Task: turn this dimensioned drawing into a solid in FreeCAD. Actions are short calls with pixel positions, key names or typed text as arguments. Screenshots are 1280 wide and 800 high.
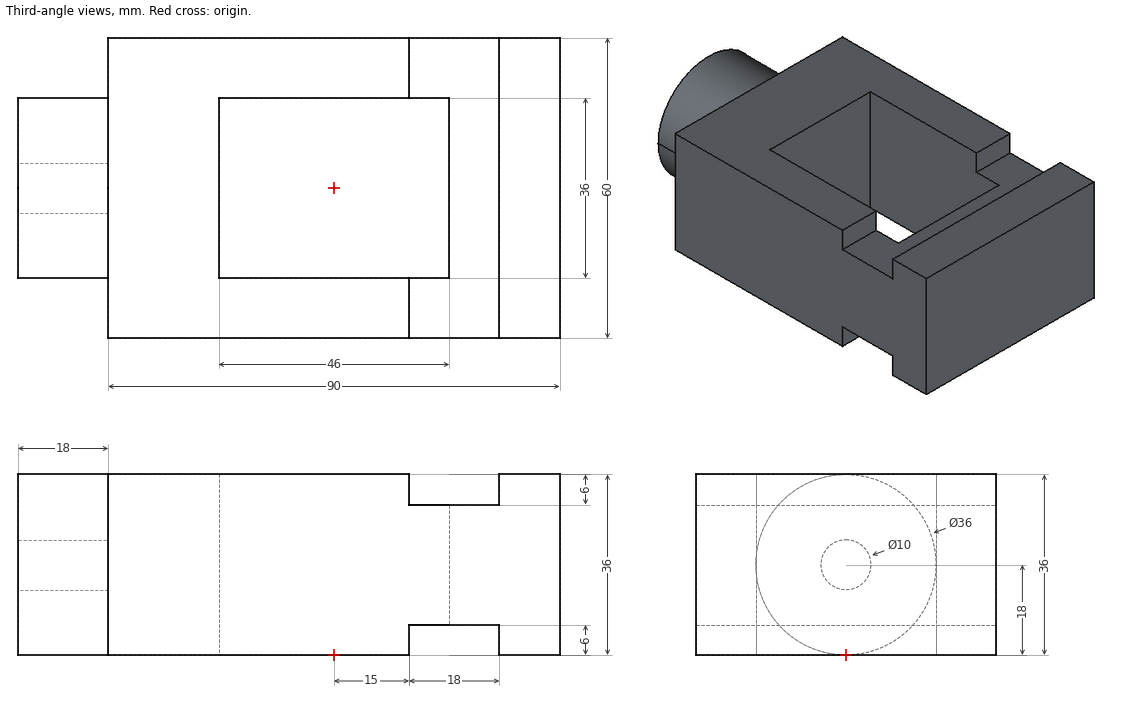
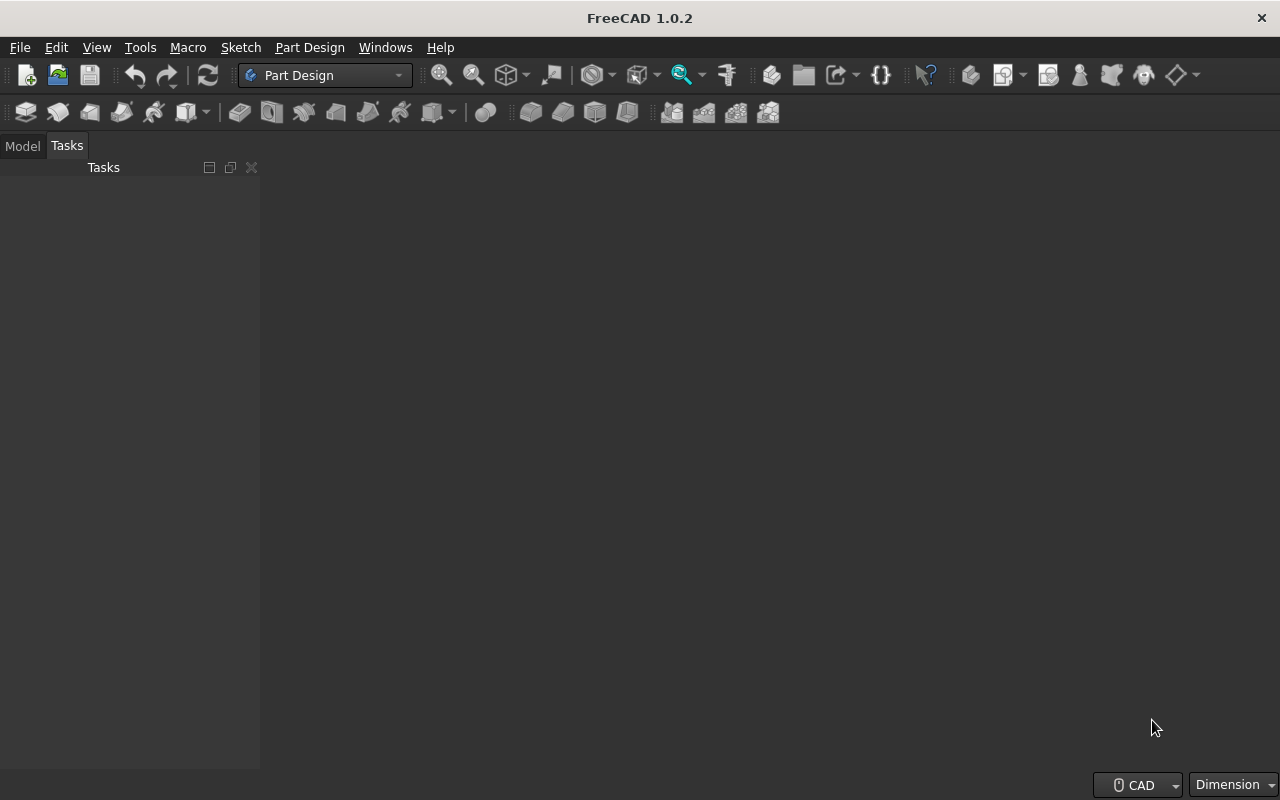
click(26, 76)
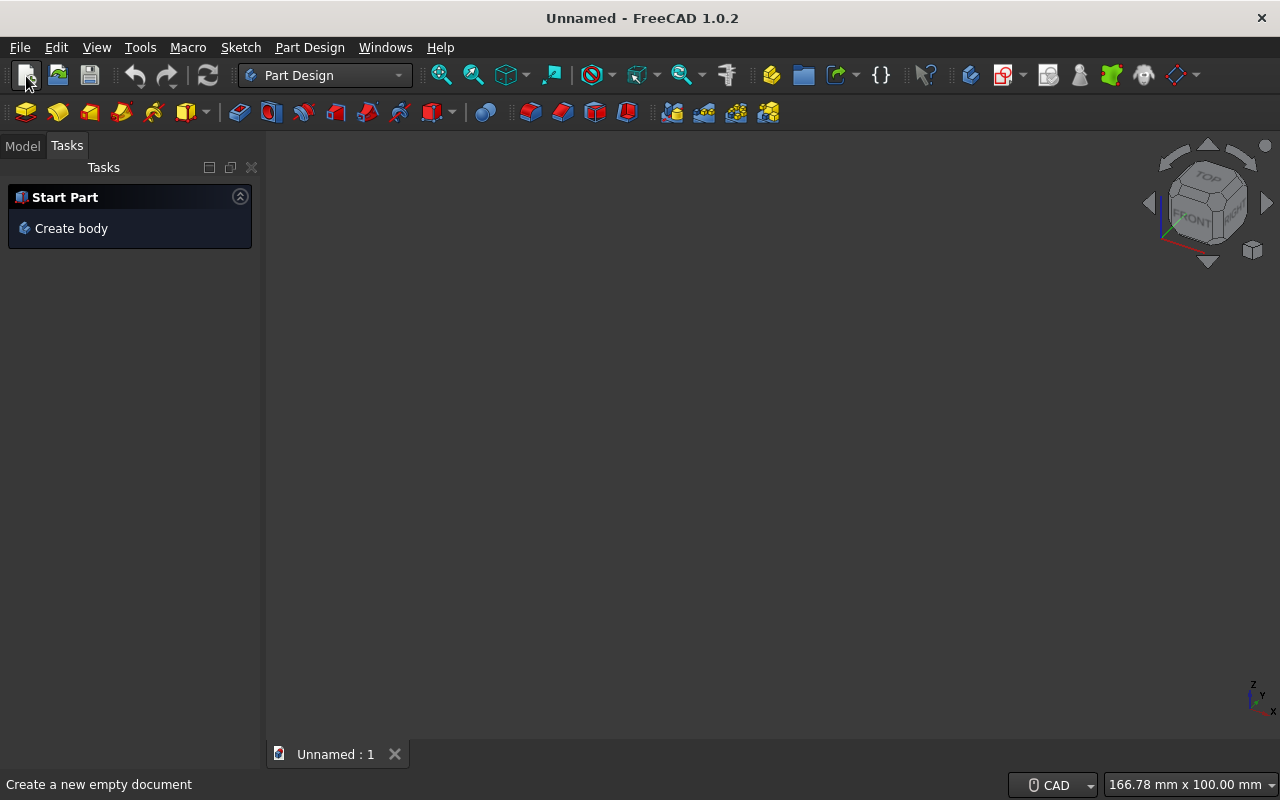
click(1004, 76)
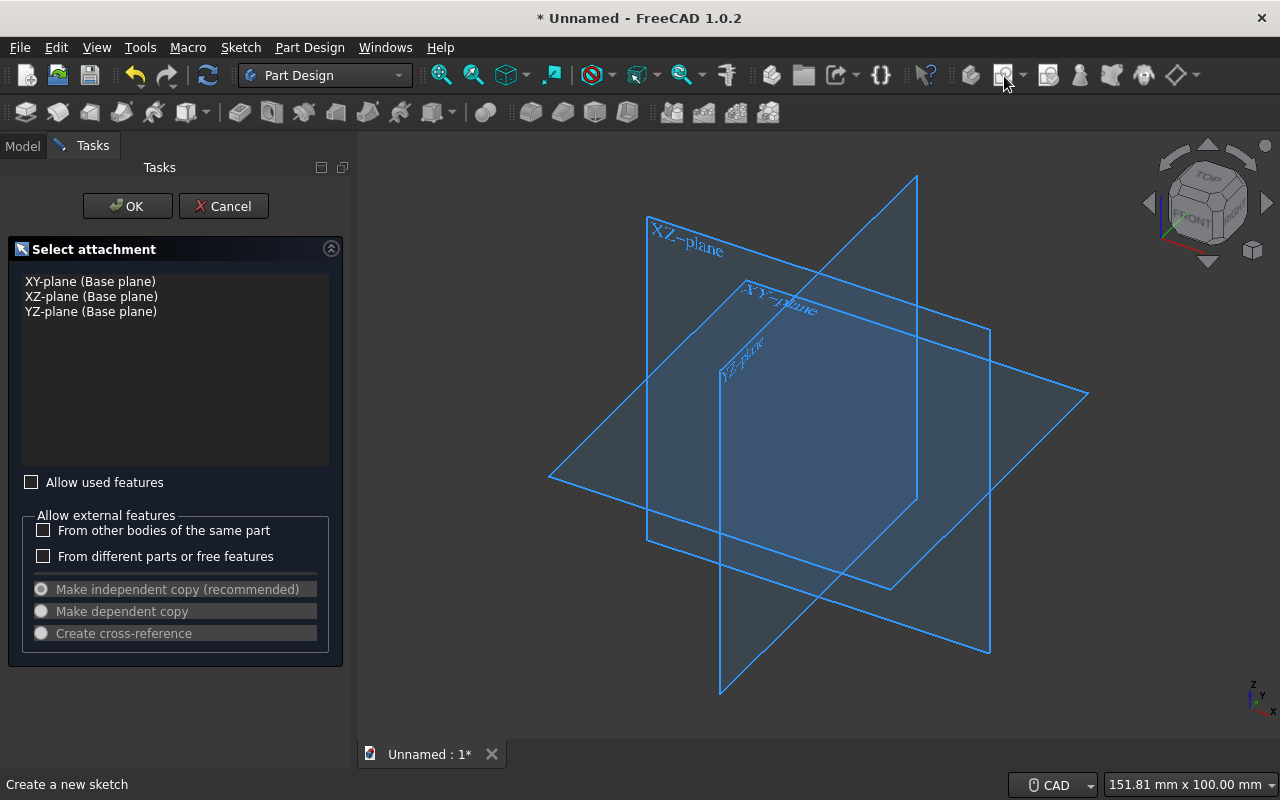
click(82, 282)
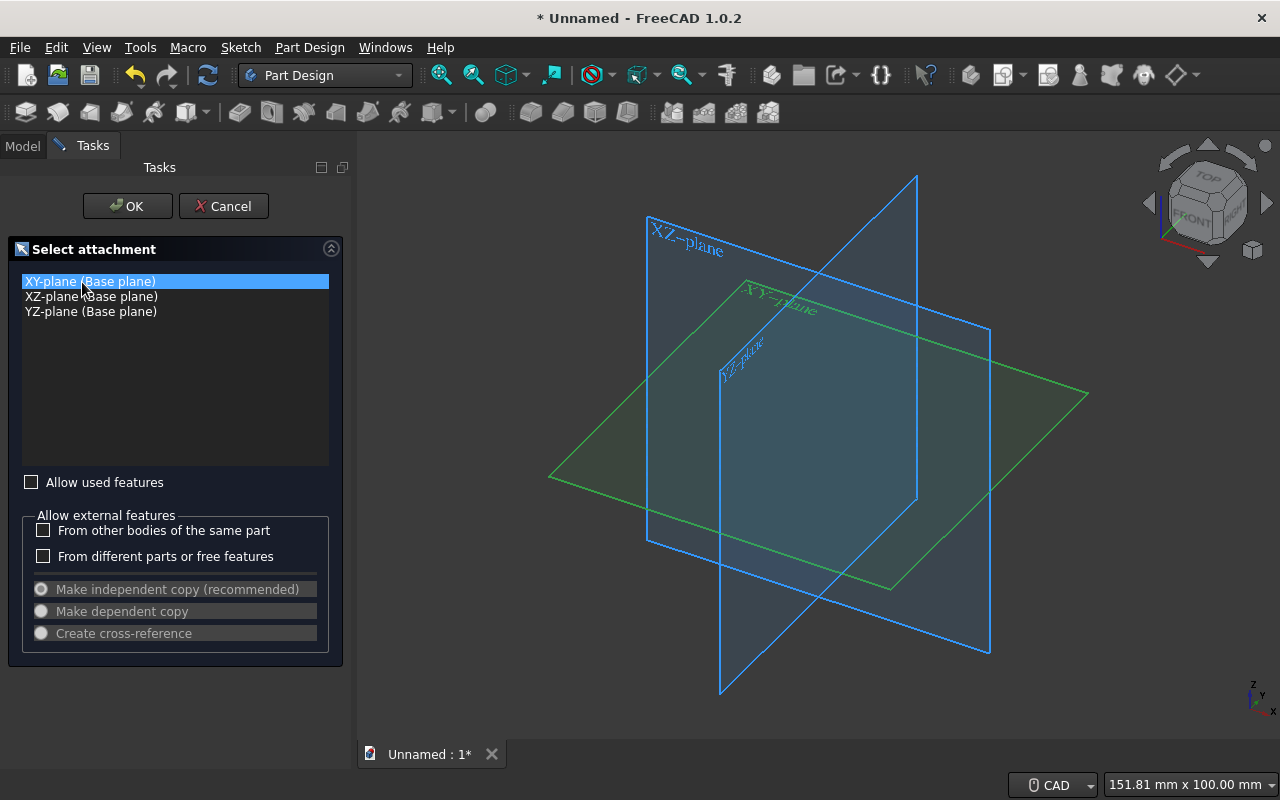
click(128, 206)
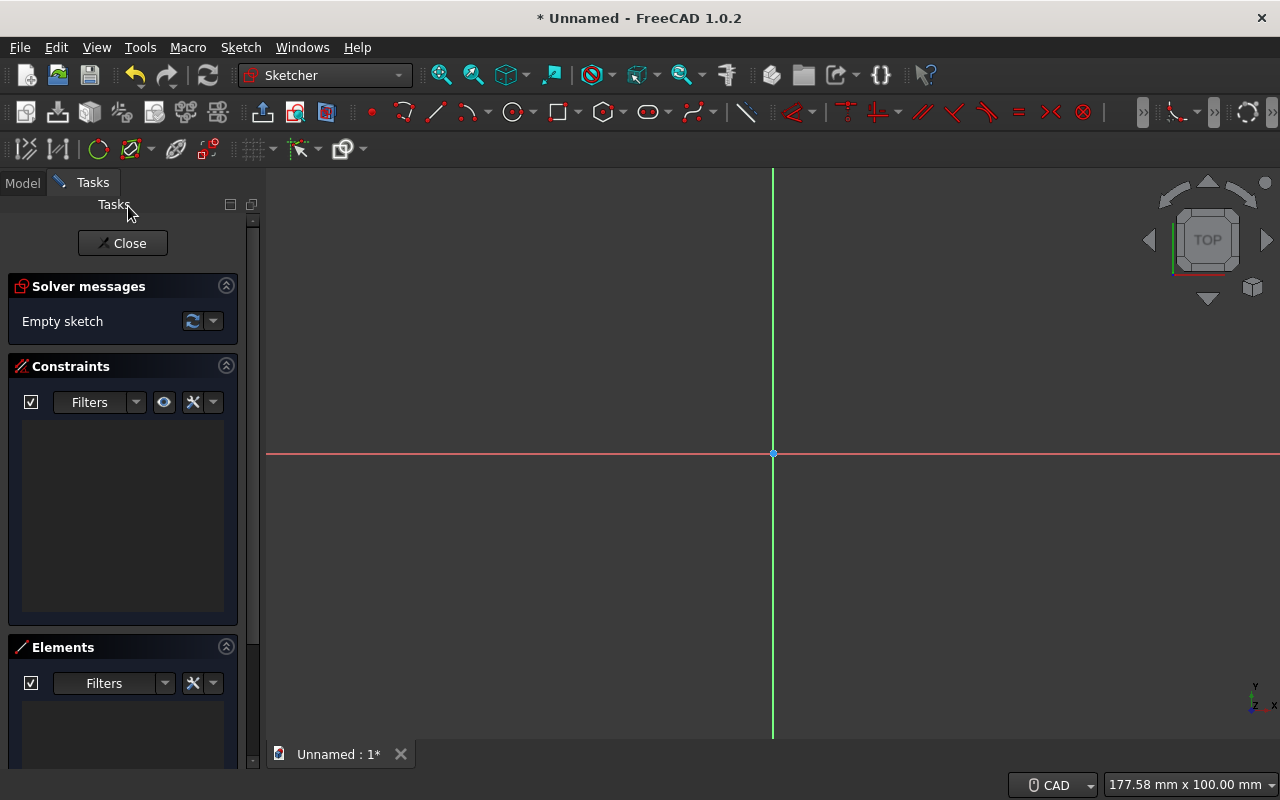
click(580, 112)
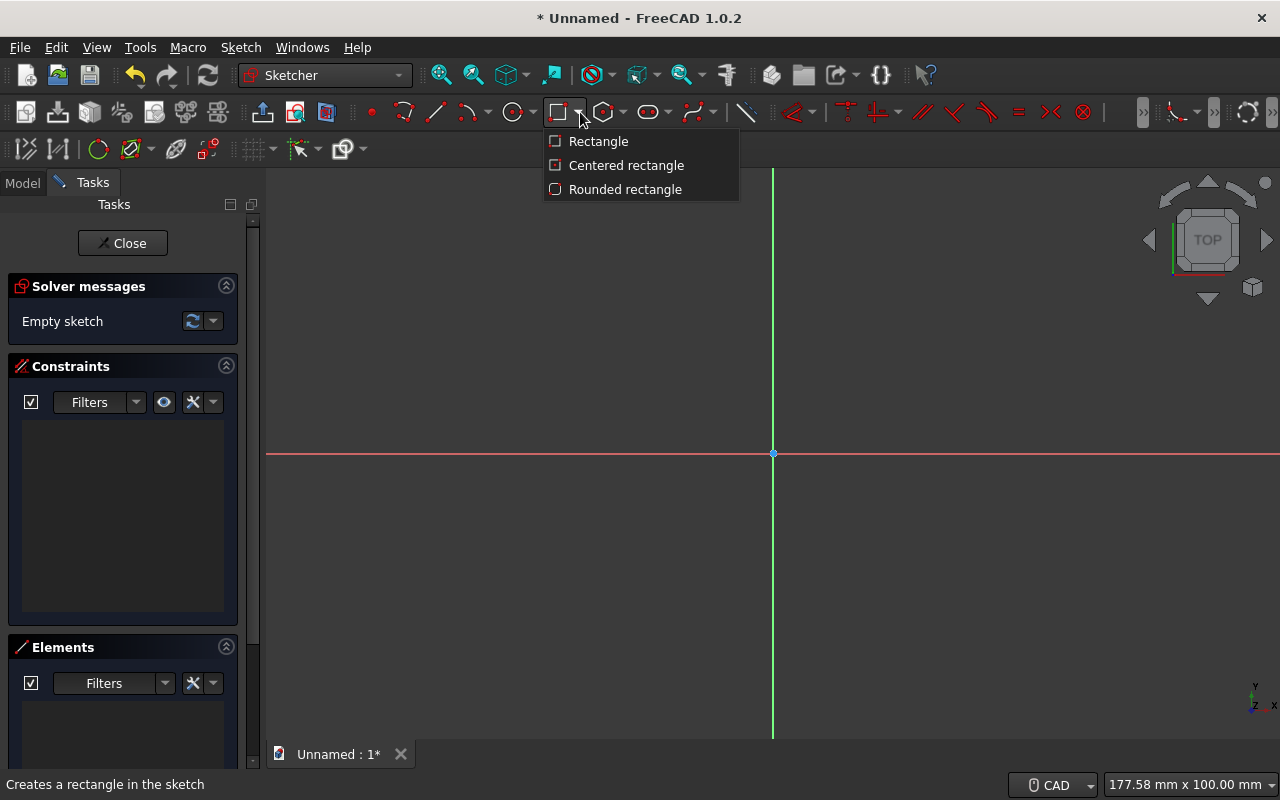
click(642, 165)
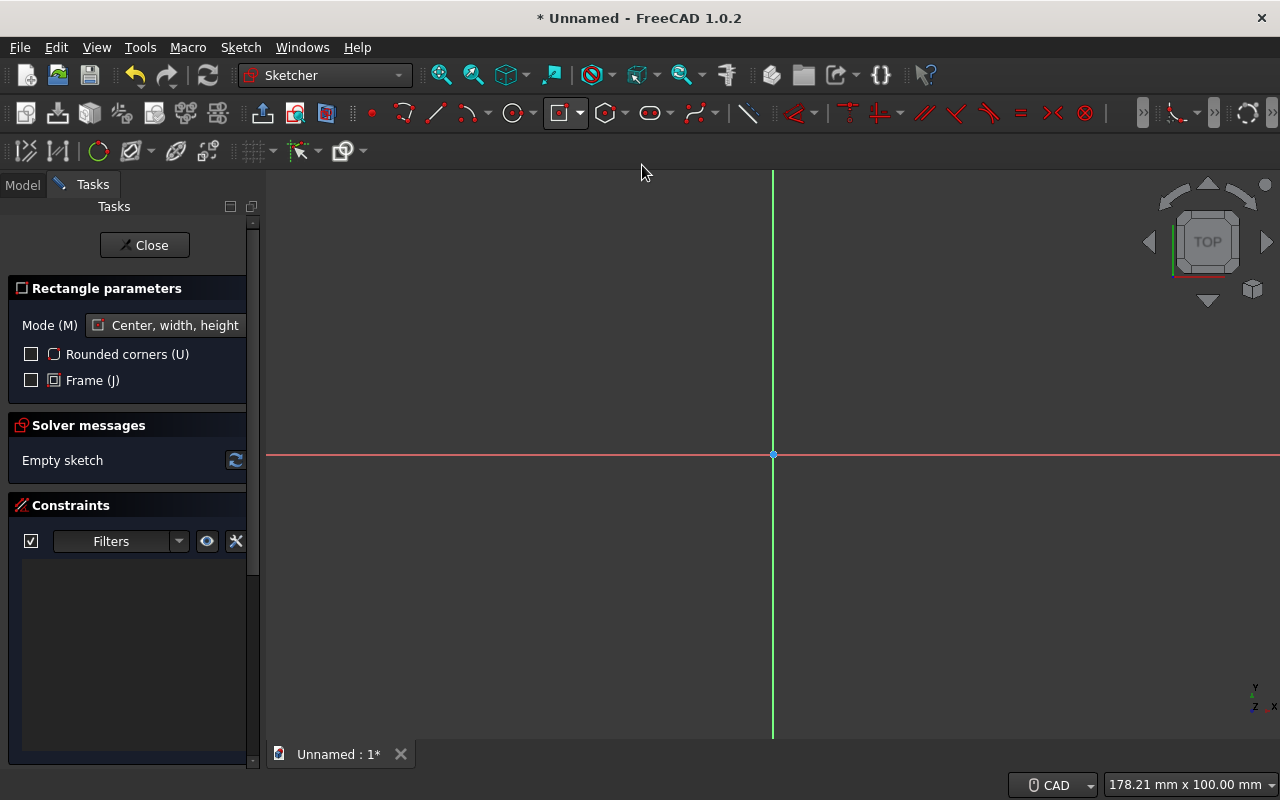
click(773, 454)
click(1029, 284)
key(Escape)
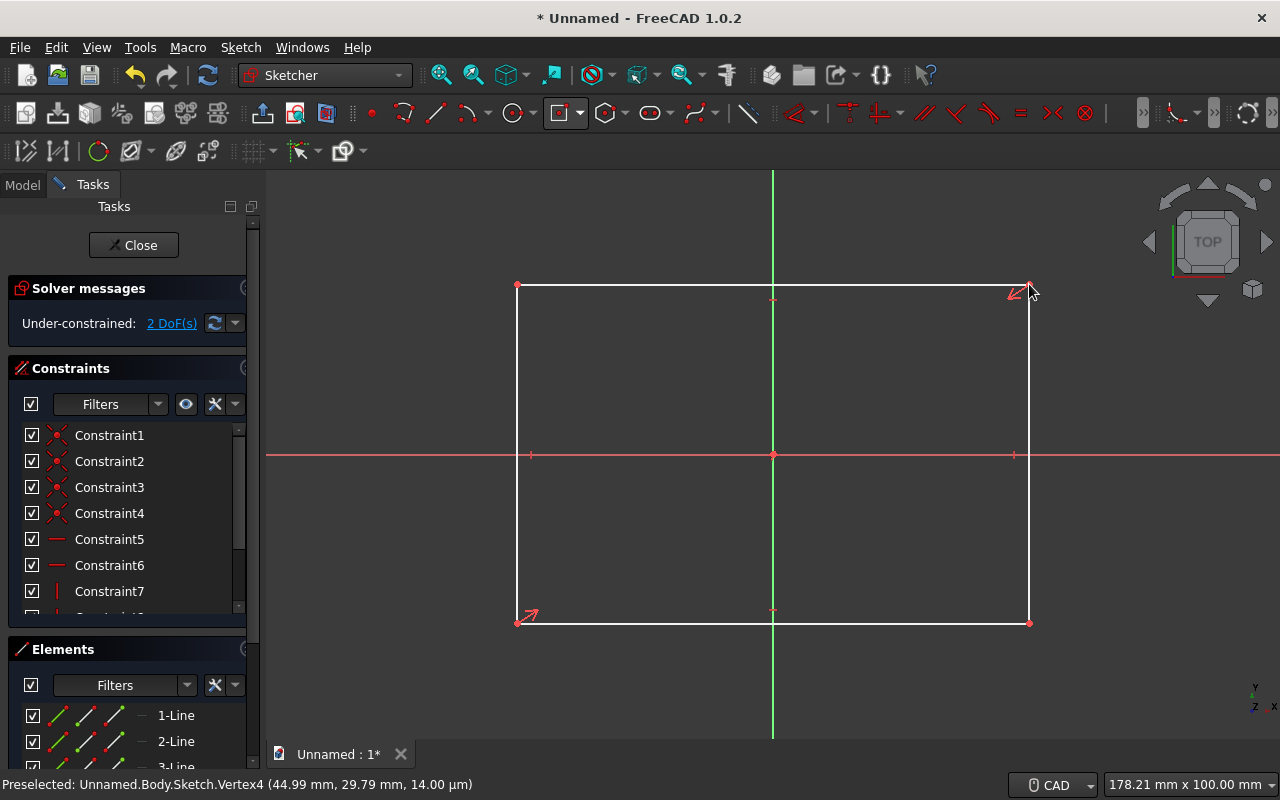
click(671, 624)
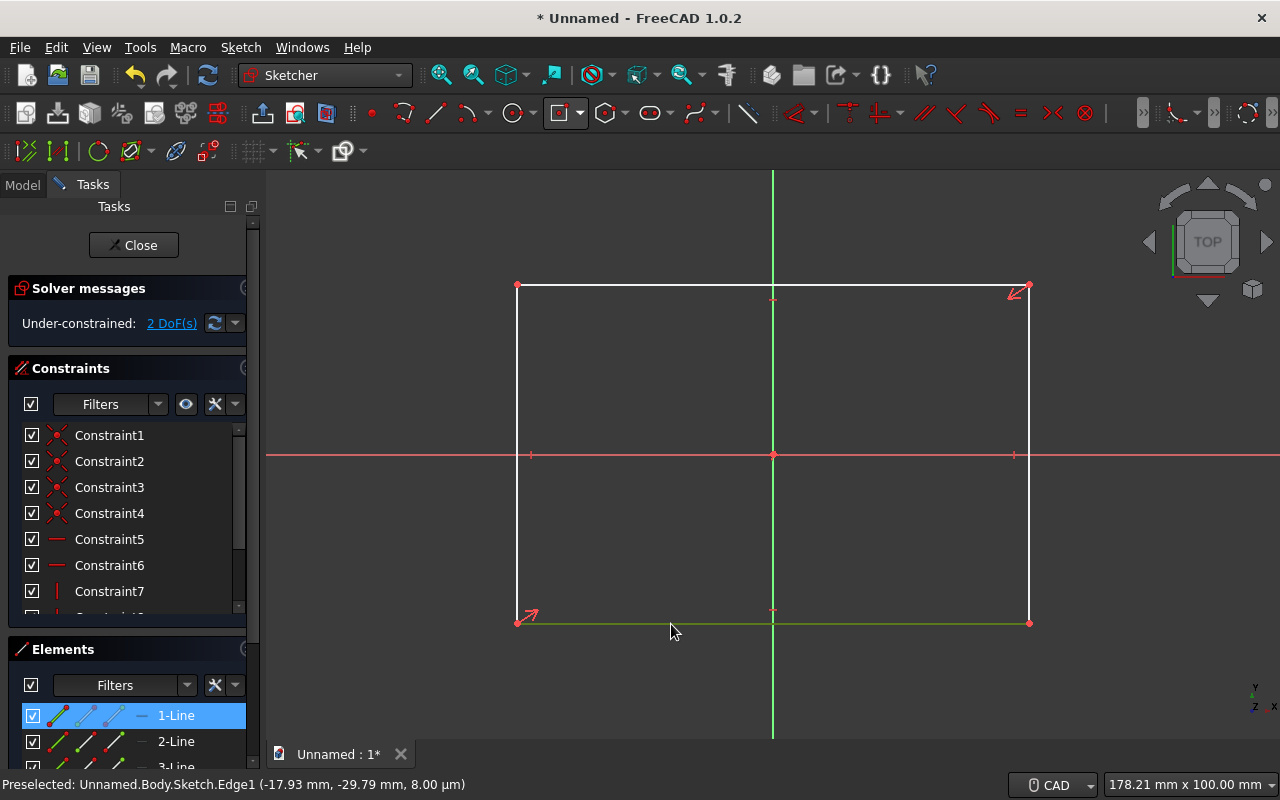
click(816, 114)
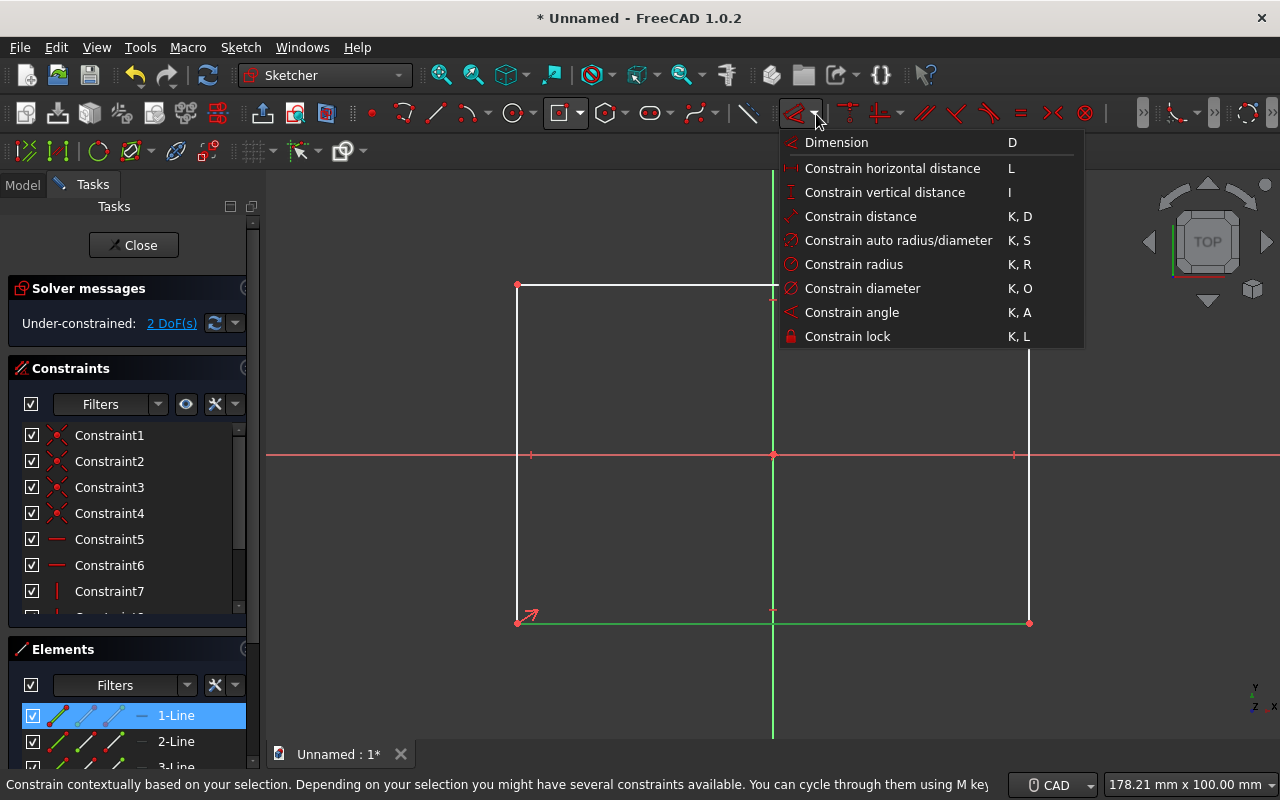
click(932, 168)